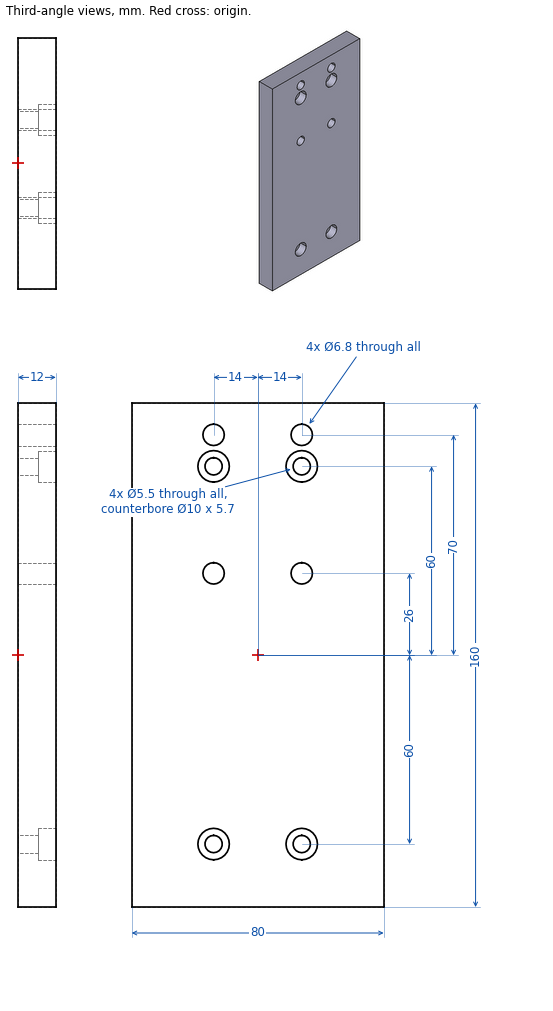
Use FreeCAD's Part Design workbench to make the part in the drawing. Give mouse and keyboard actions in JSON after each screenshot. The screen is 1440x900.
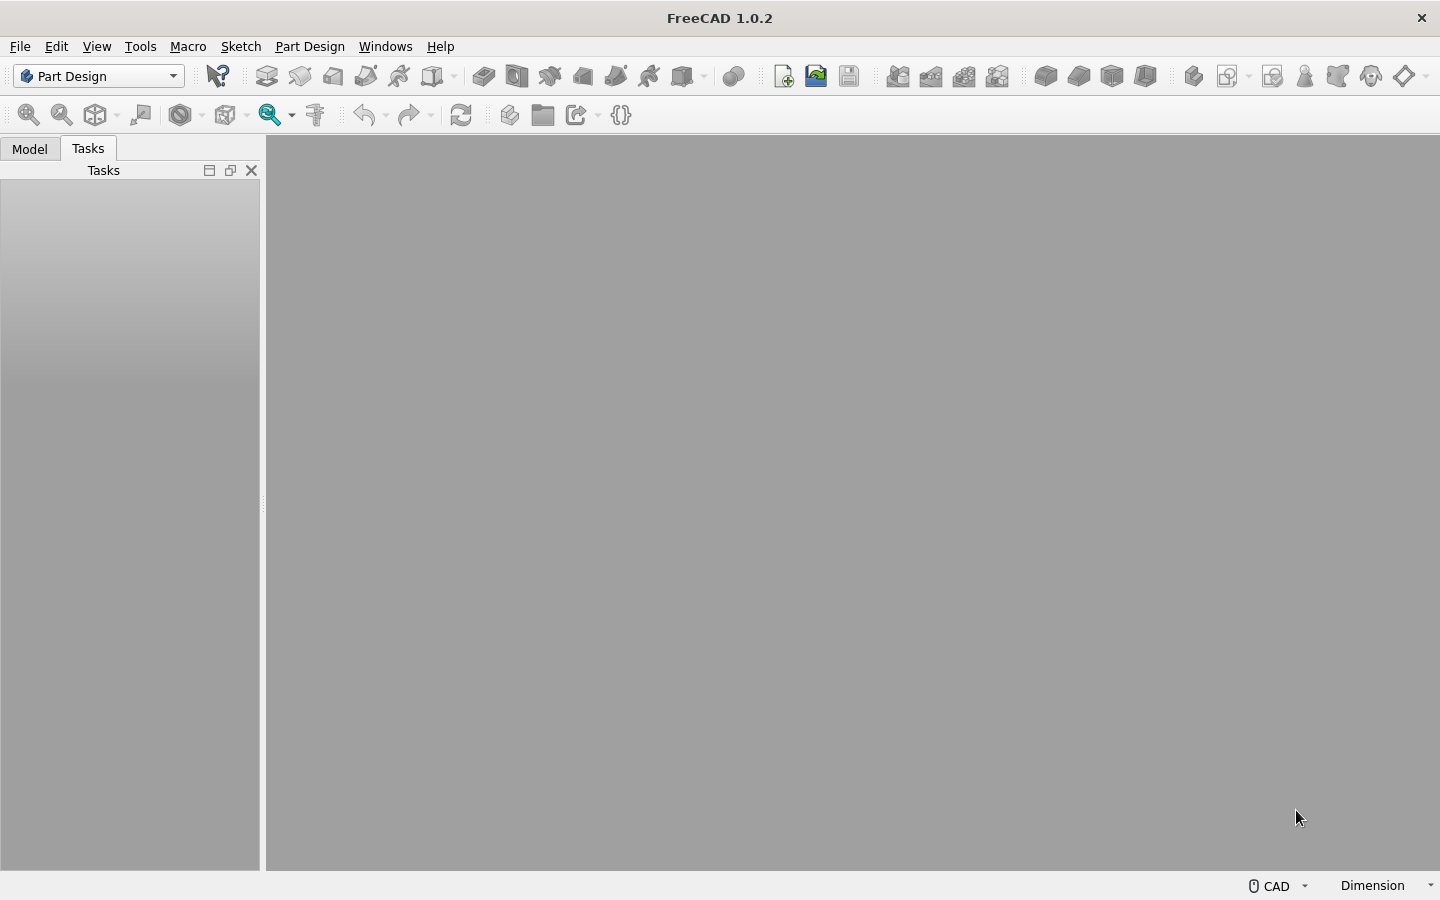
{"action": "left_click", "coordinate": [783, 76]}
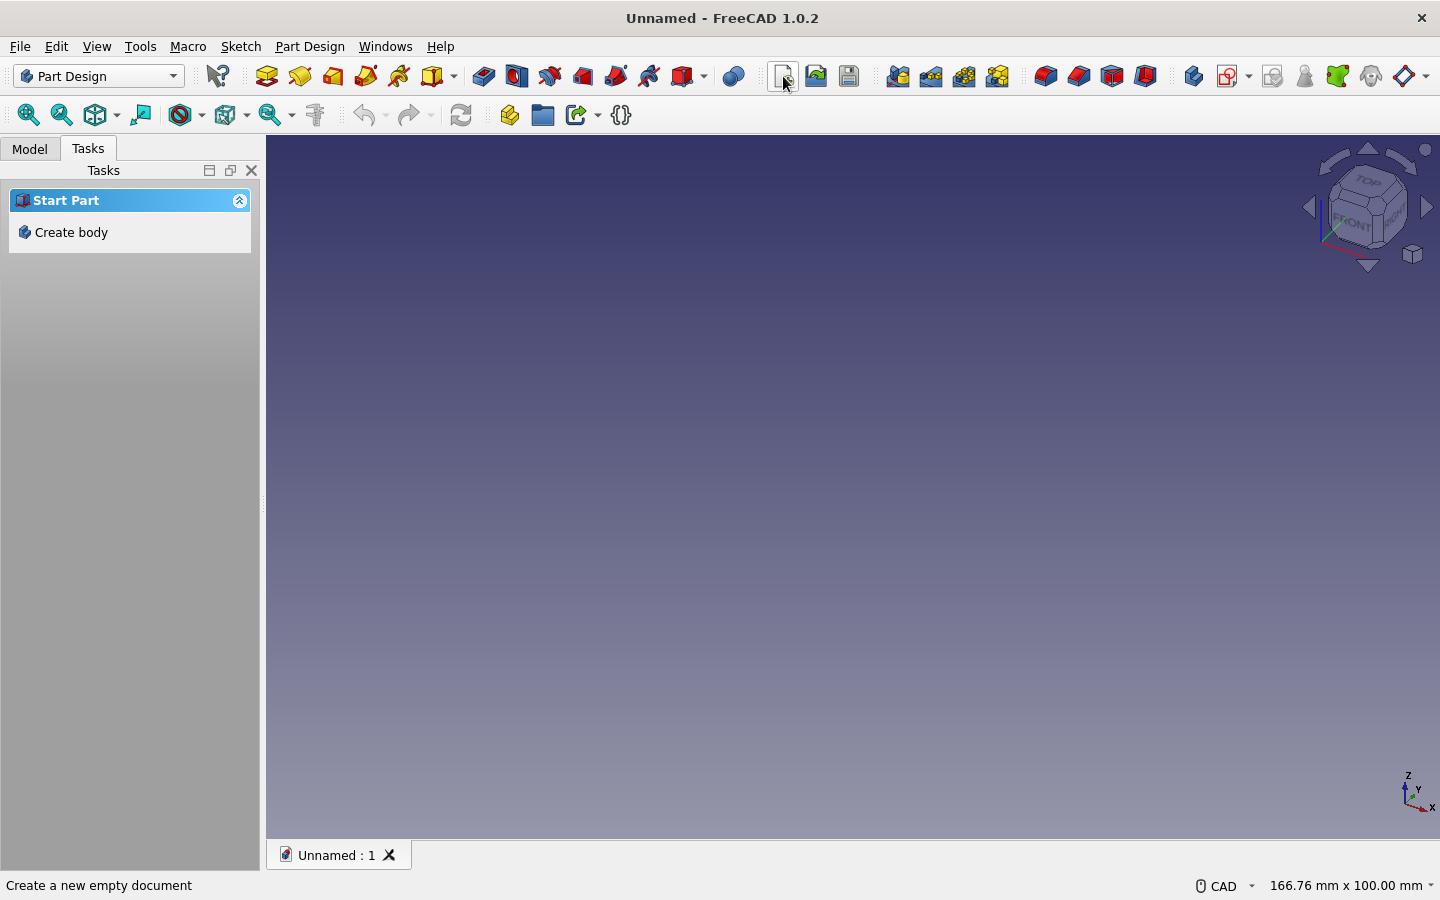
{"action": "left_click", "coordinate": [1226, 76]}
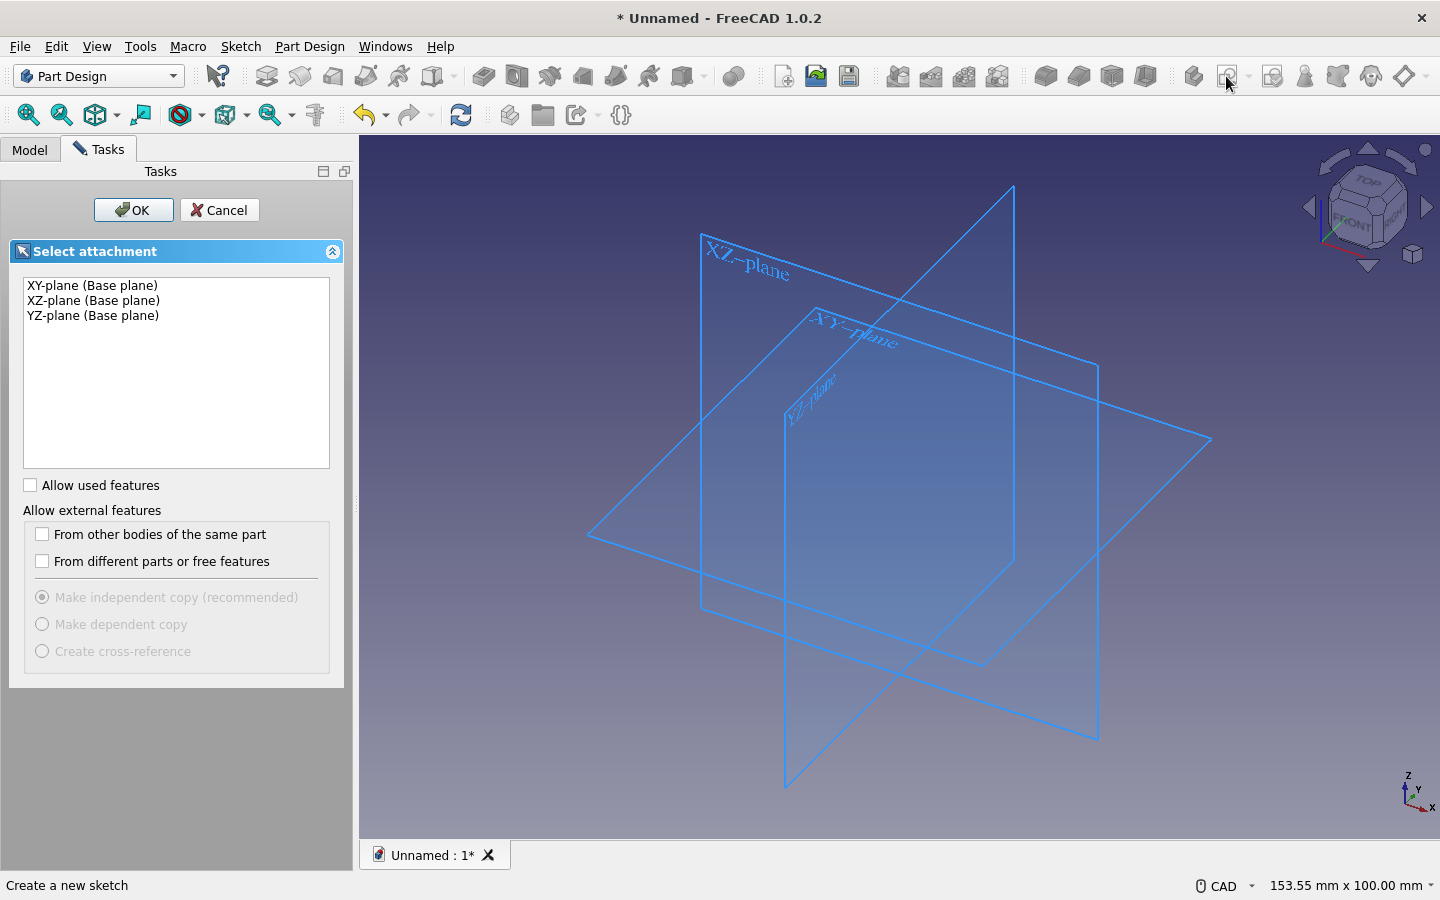
{"action": "left_click", "coordinate": [84, 316]}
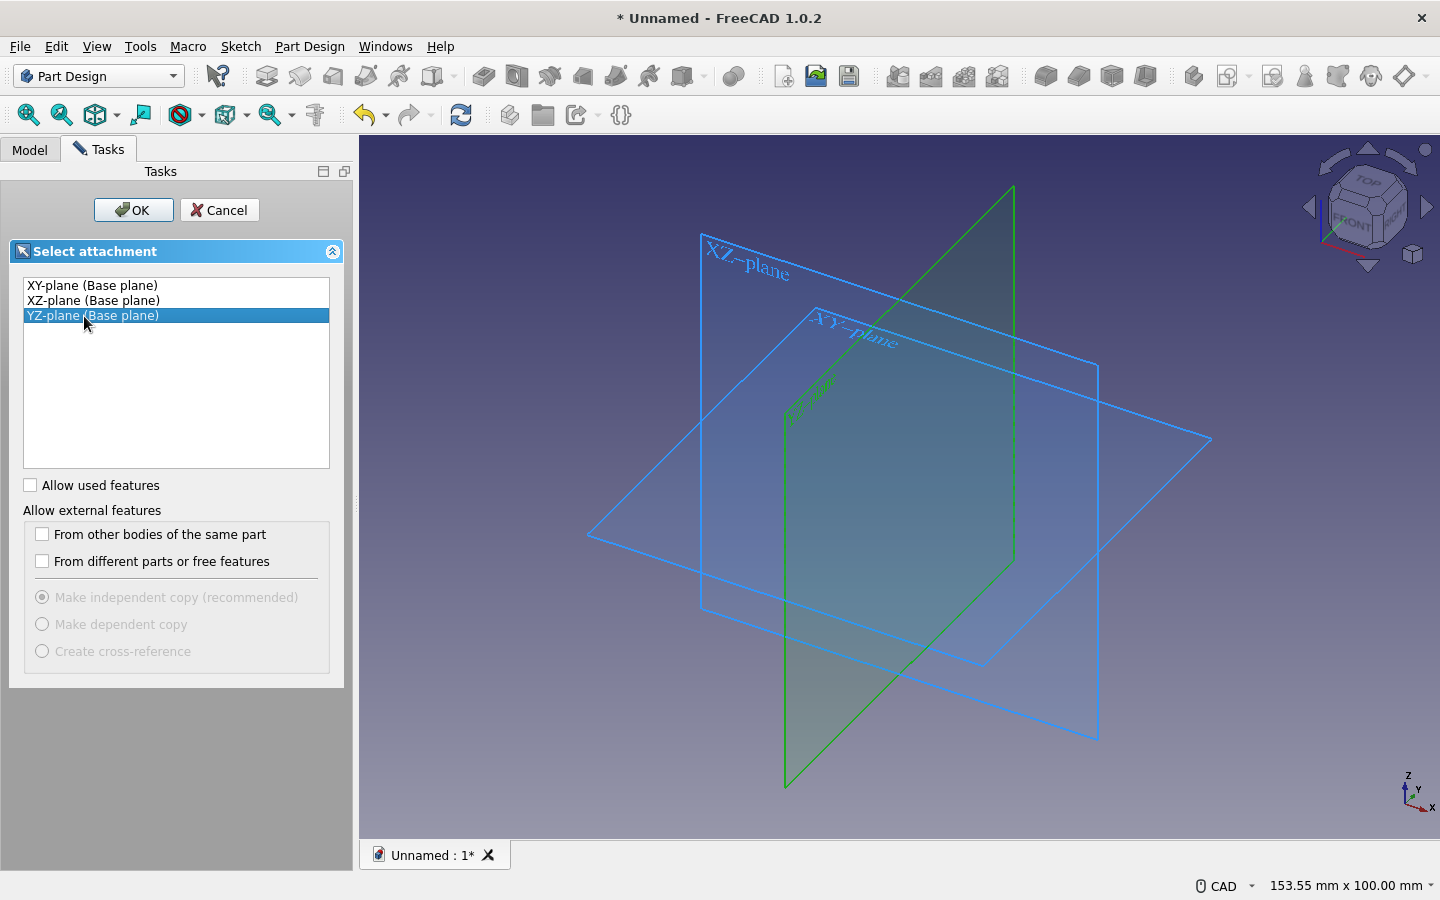
{"action": "left_click", "coordinate": [134, 210]}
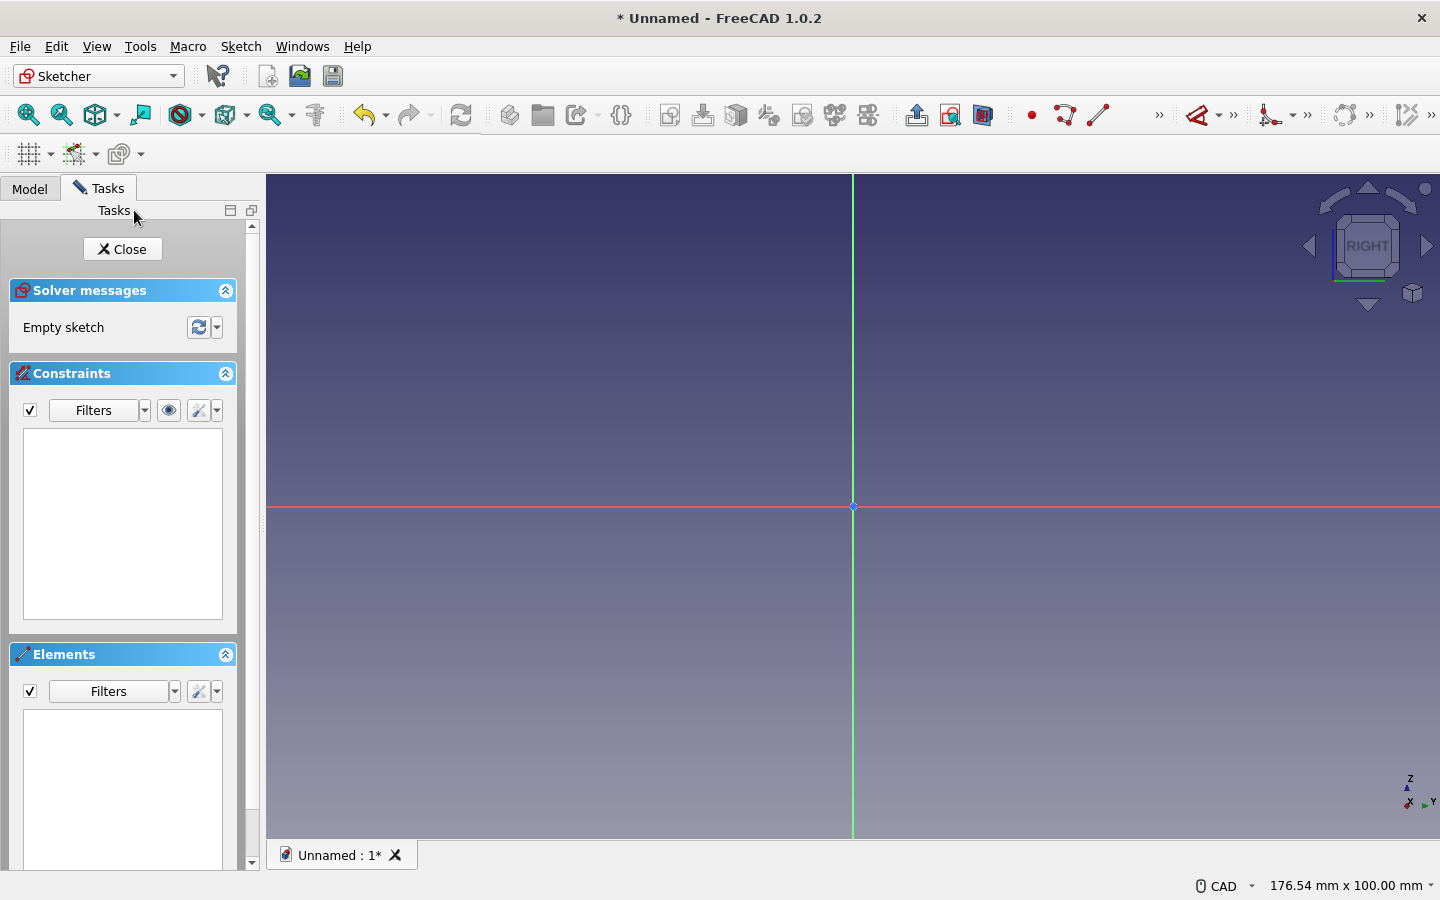
{"action": "scroll", "coordinate": [745, 506], "scroll_direction": "down", "scroll_amount": 5}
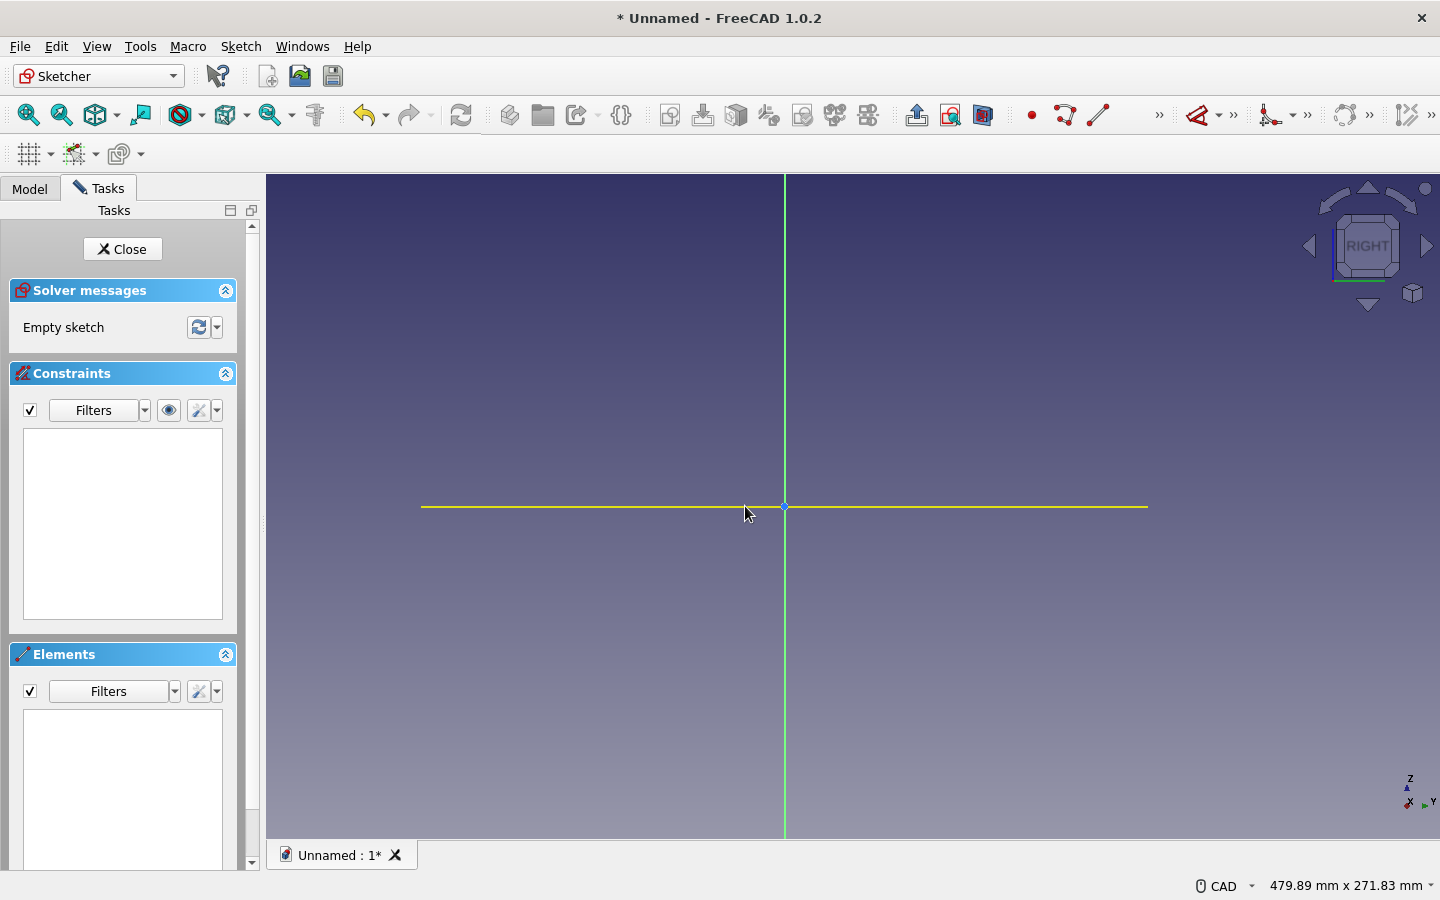
{"action": "key", "text": "g v"}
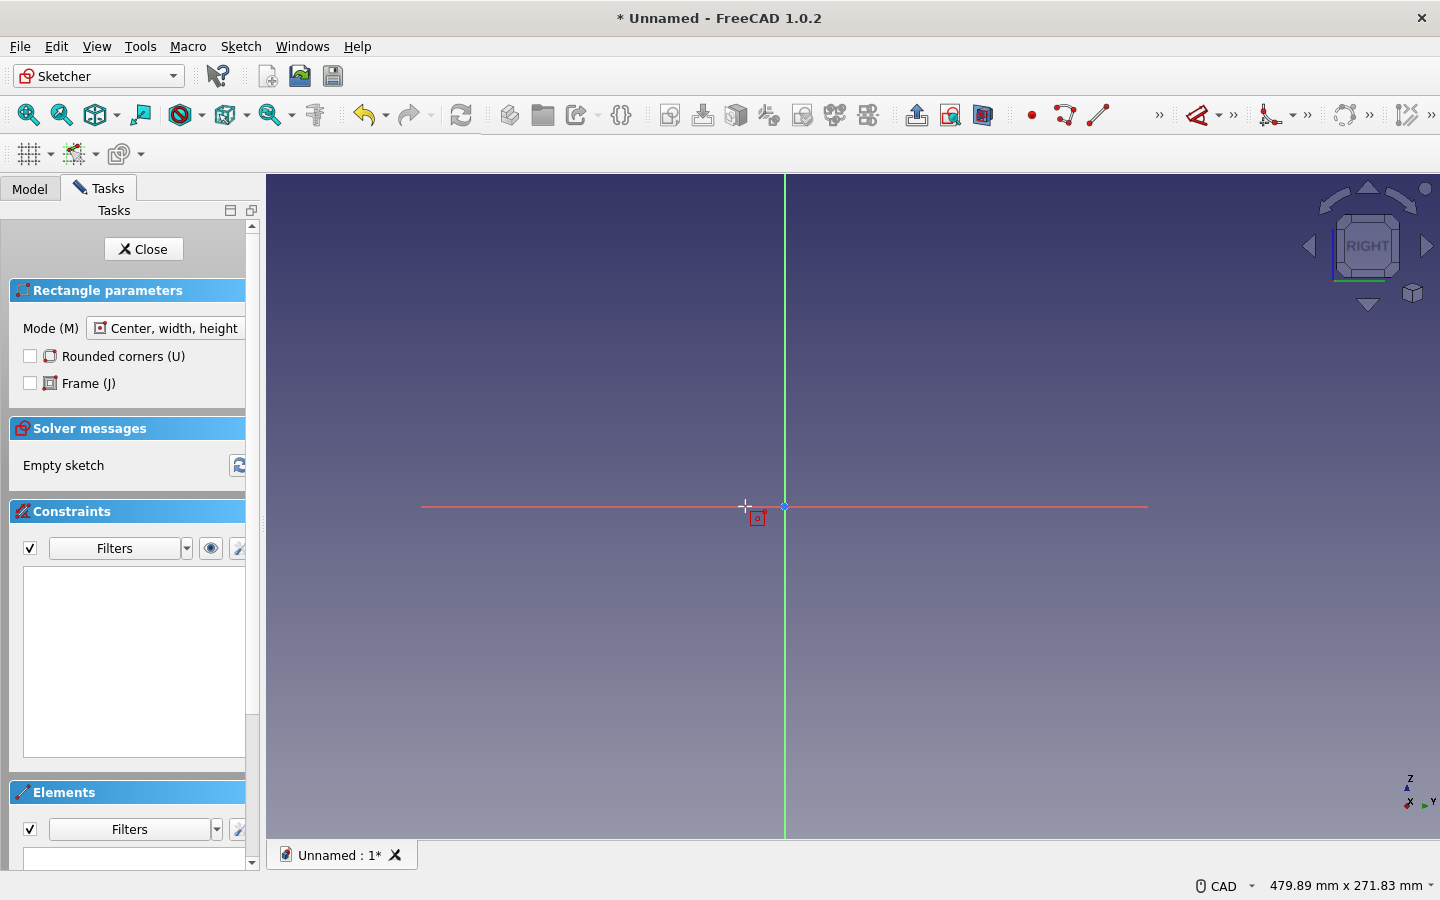
{"action": "left_click", "coordinate": [785, 506]}
{"action": "left_click", "coordinate": [883, 311]}
{"action": "key", "text": "Escape"}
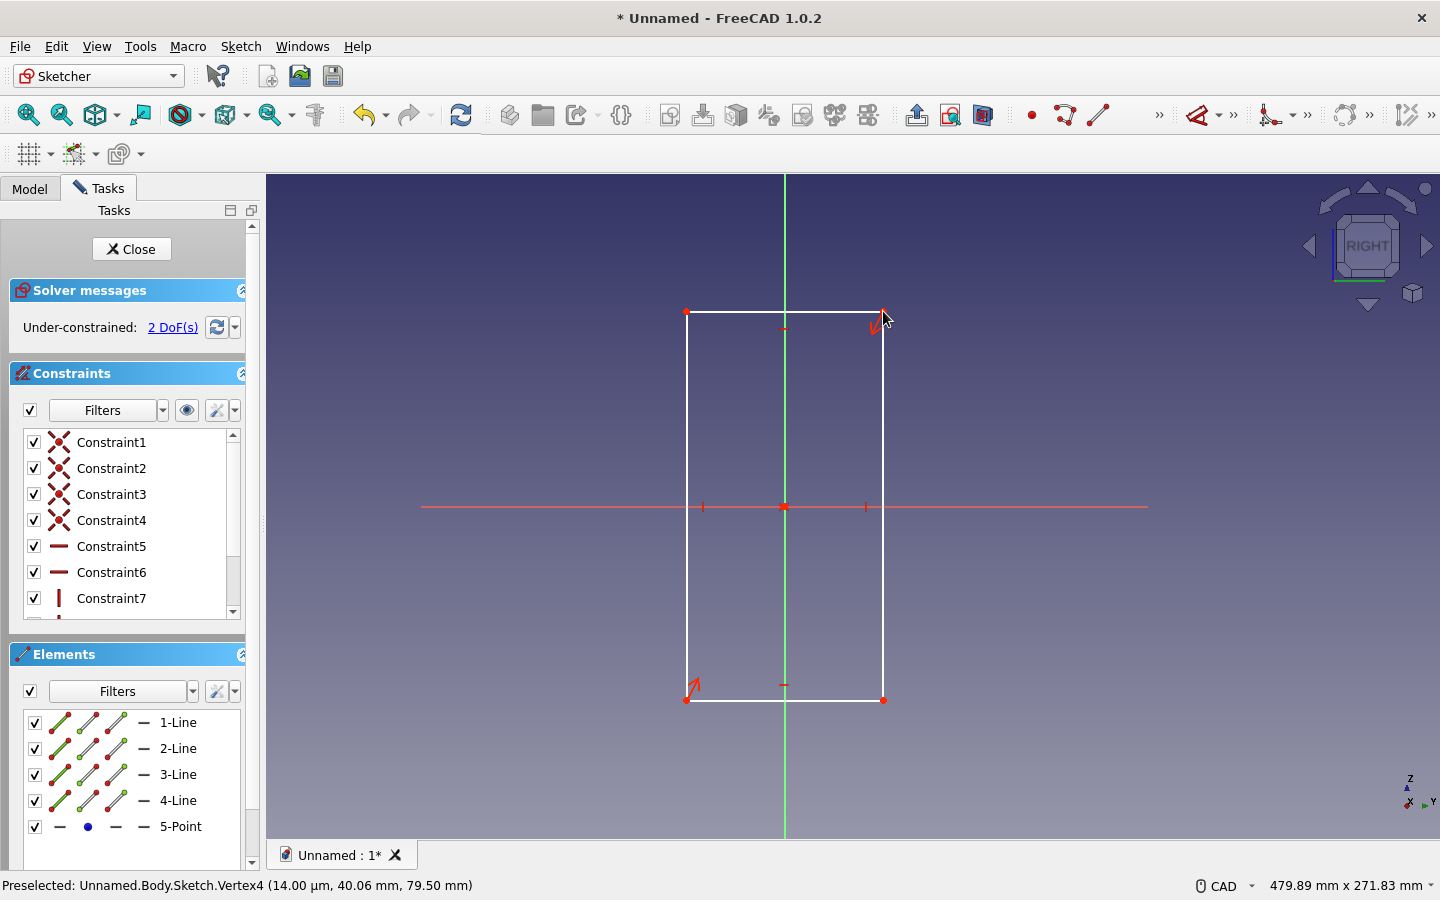
{"action": "left_click", "coordinate": [1196, 116]}